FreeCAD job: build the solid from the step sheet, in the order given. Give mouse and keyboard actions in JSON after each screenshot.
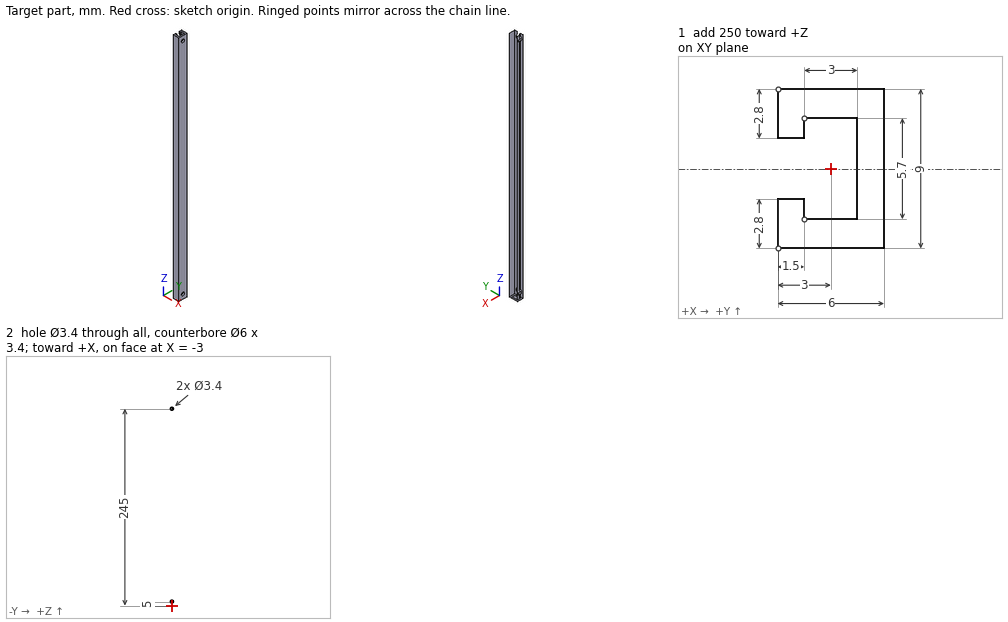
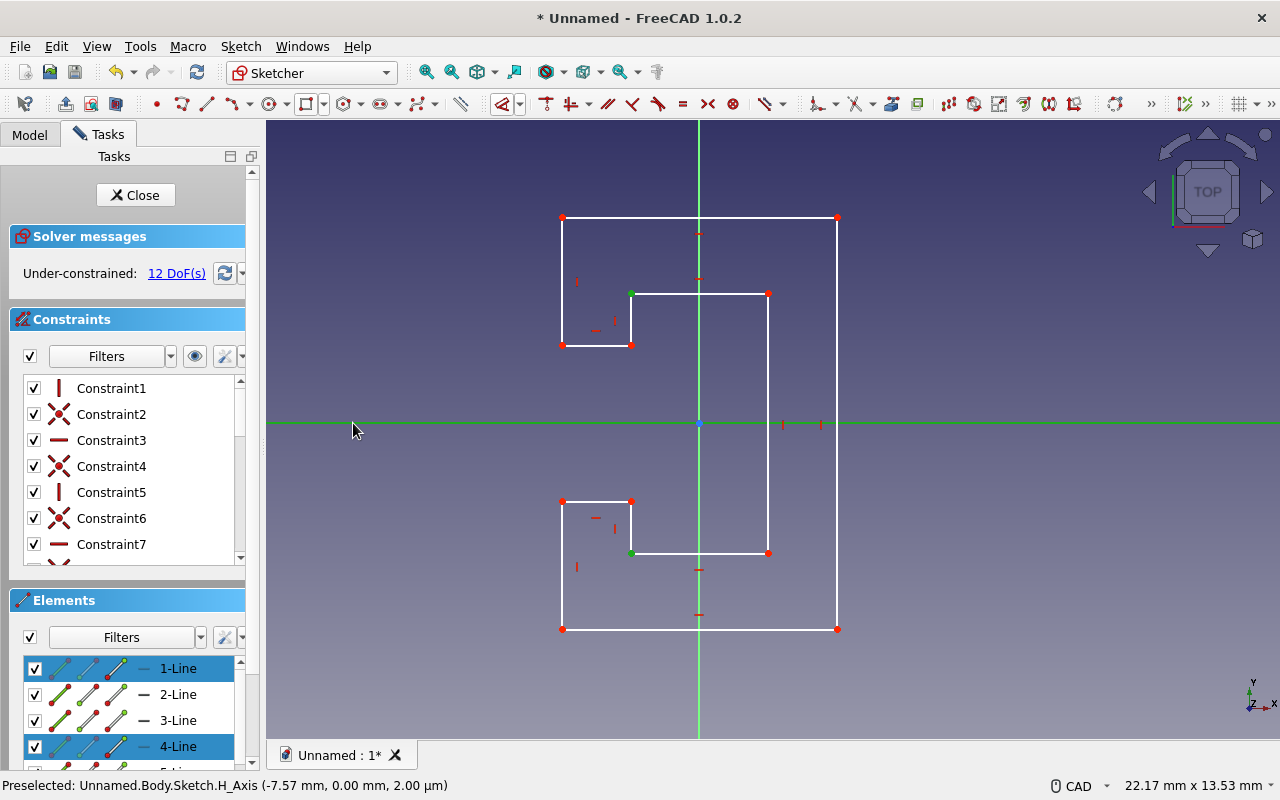
{"action": "left_click", "coordinate": [708, 104]}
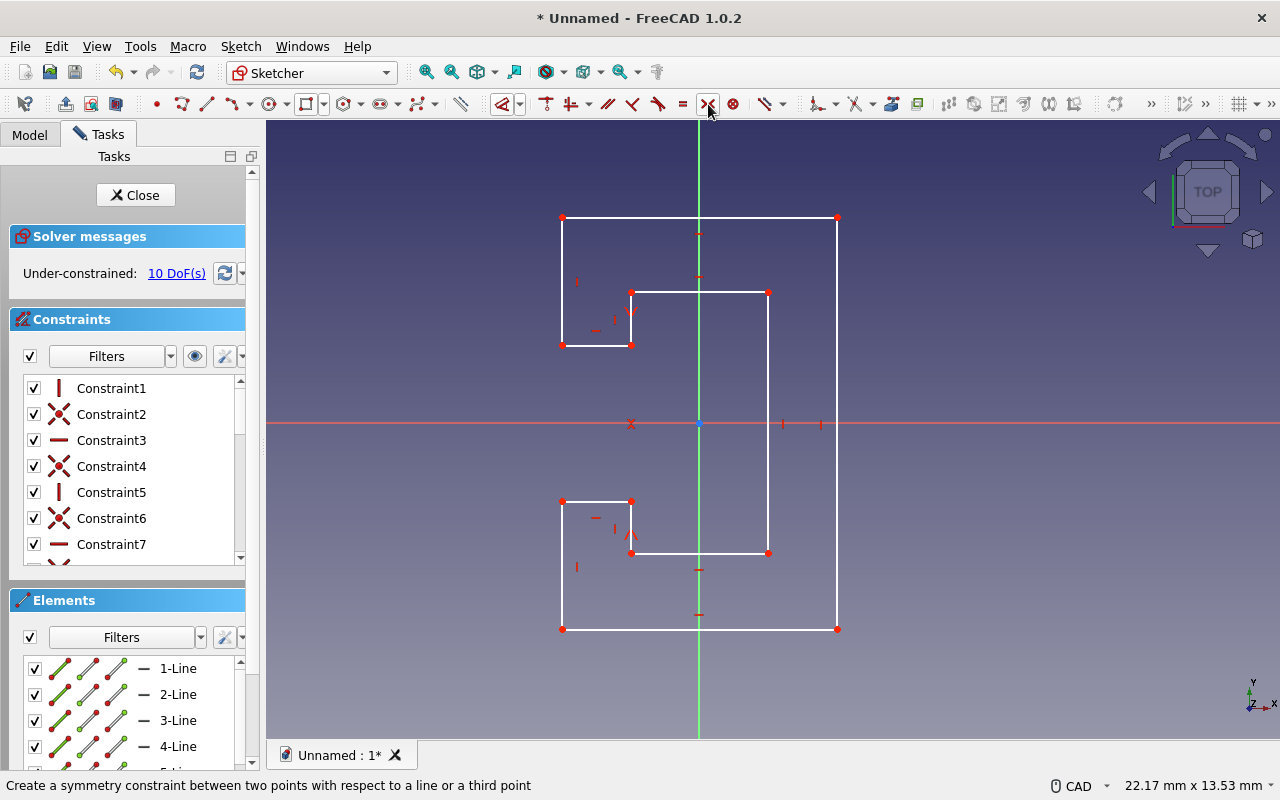
{"action": "left_click", "coordinate": [562, 630]}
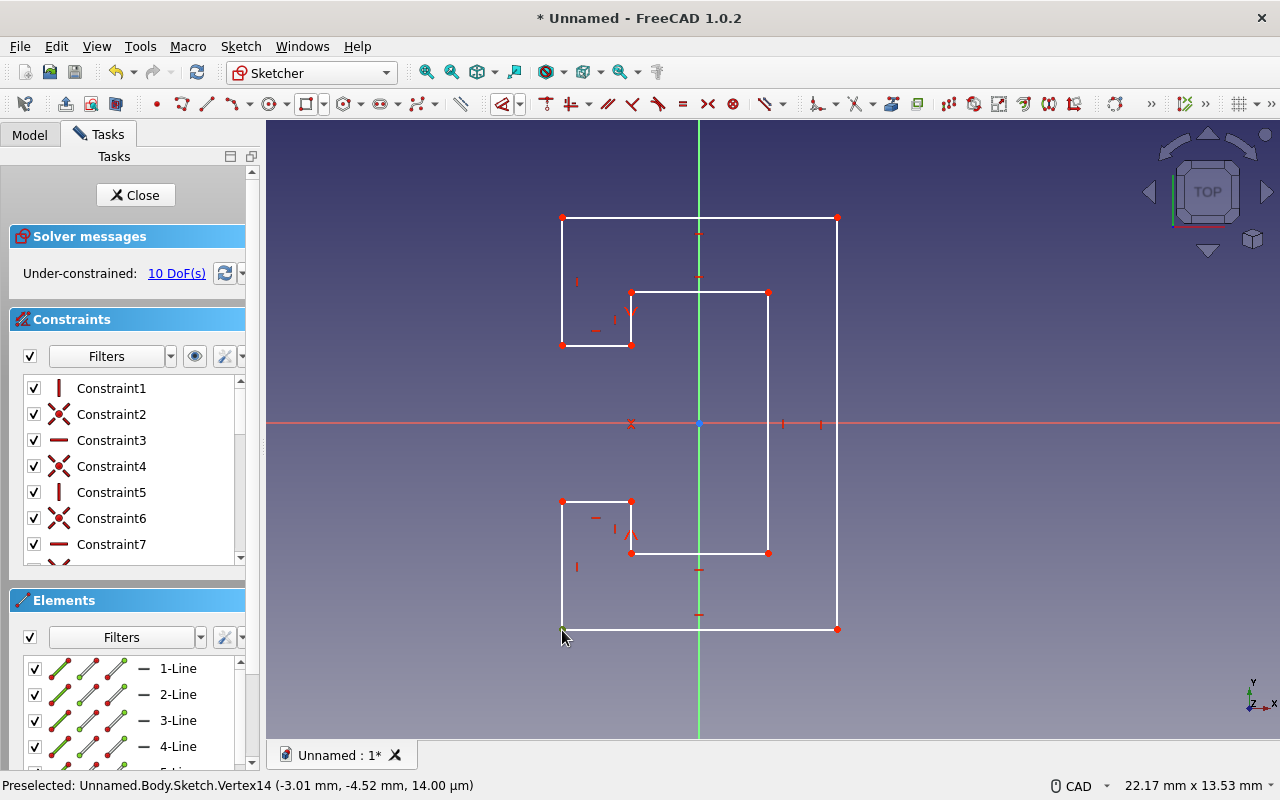
{"action": "left_click", "coordinate": [562, 218]}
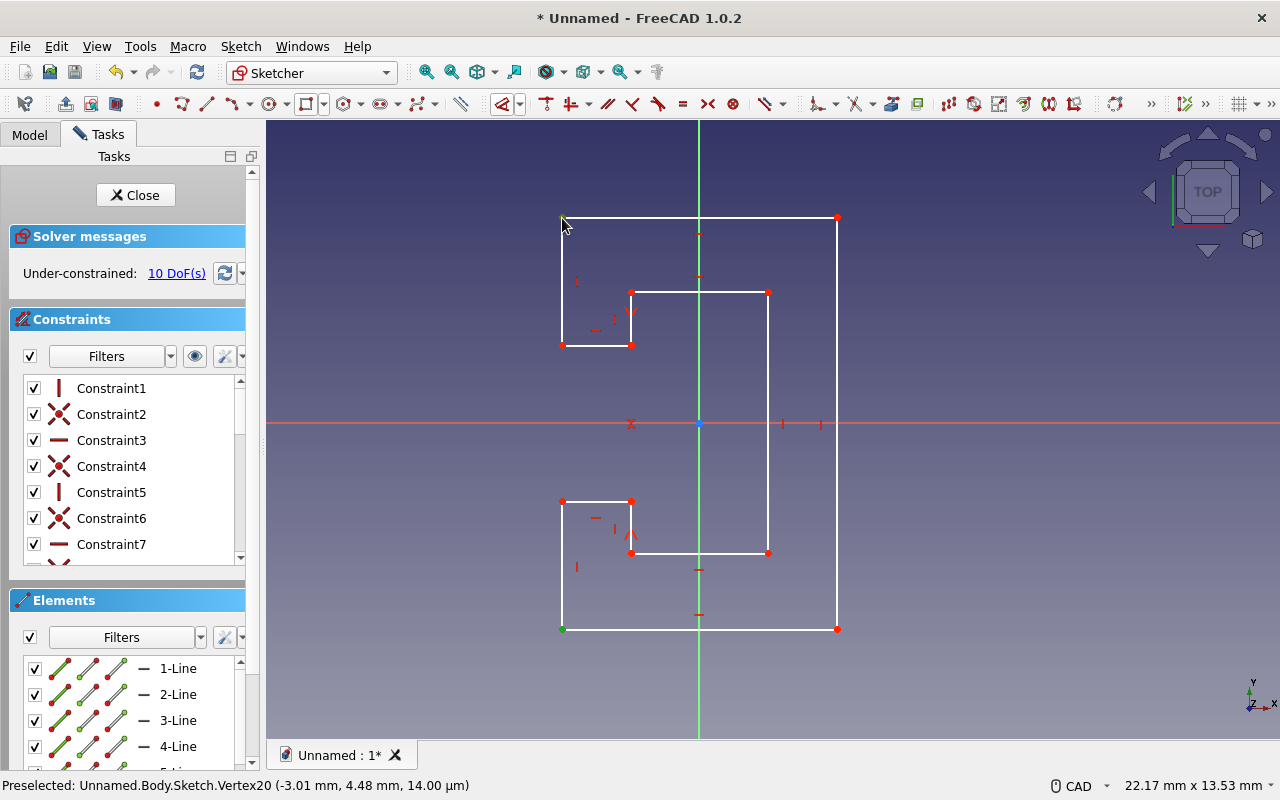
{"action": "left_click", "coordinate": [353, 423]}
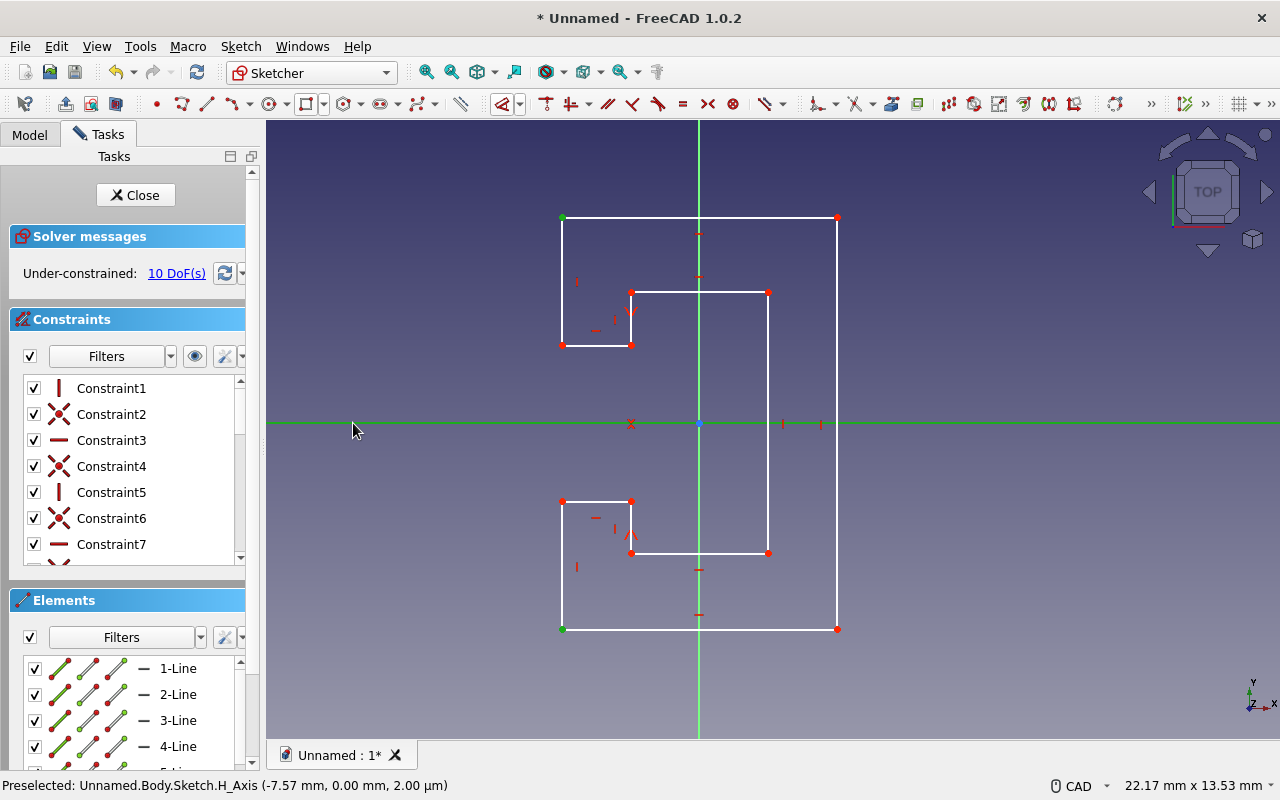
{"action": "left_click", "coordinate": [708, 104]}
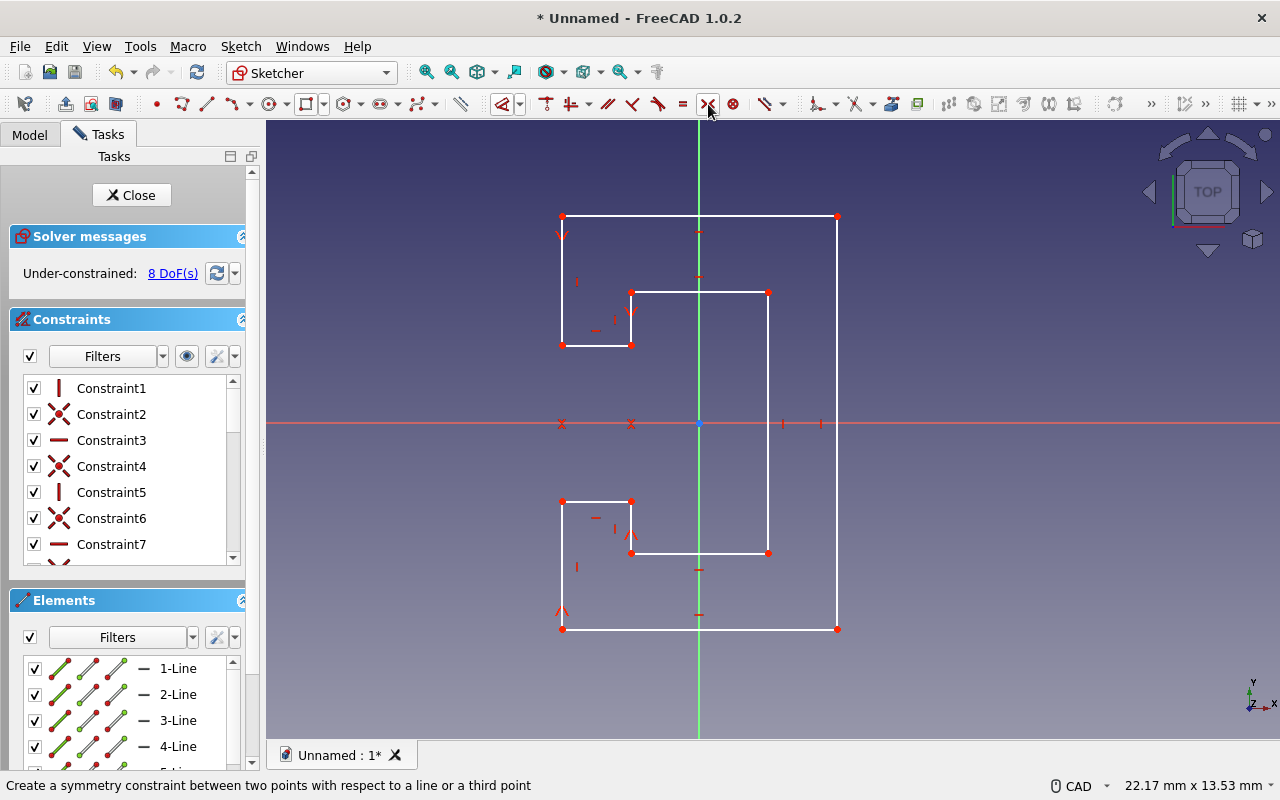
{"action": "key", "text": "d"}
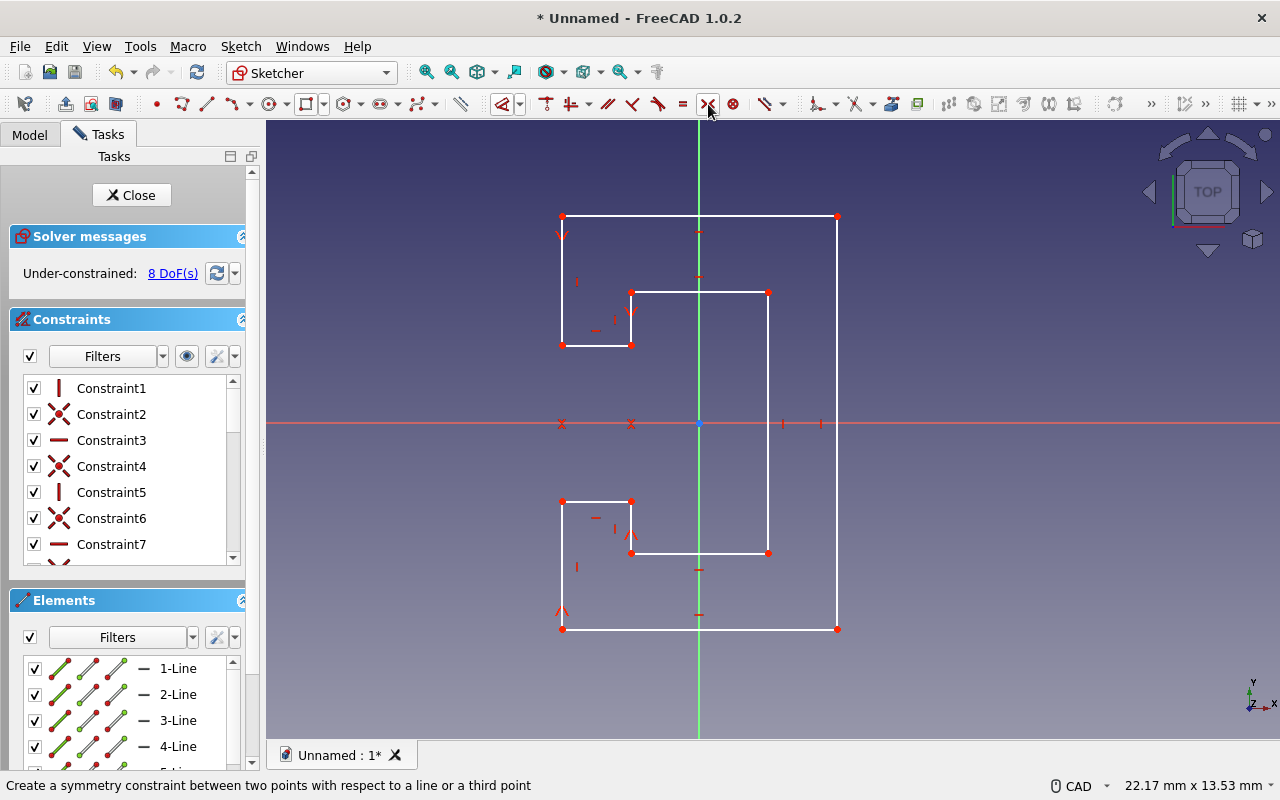
{"action": "left_click", "coordinate": [672, 292]}
{"action": "left_click", "coordinate": [668, 258]}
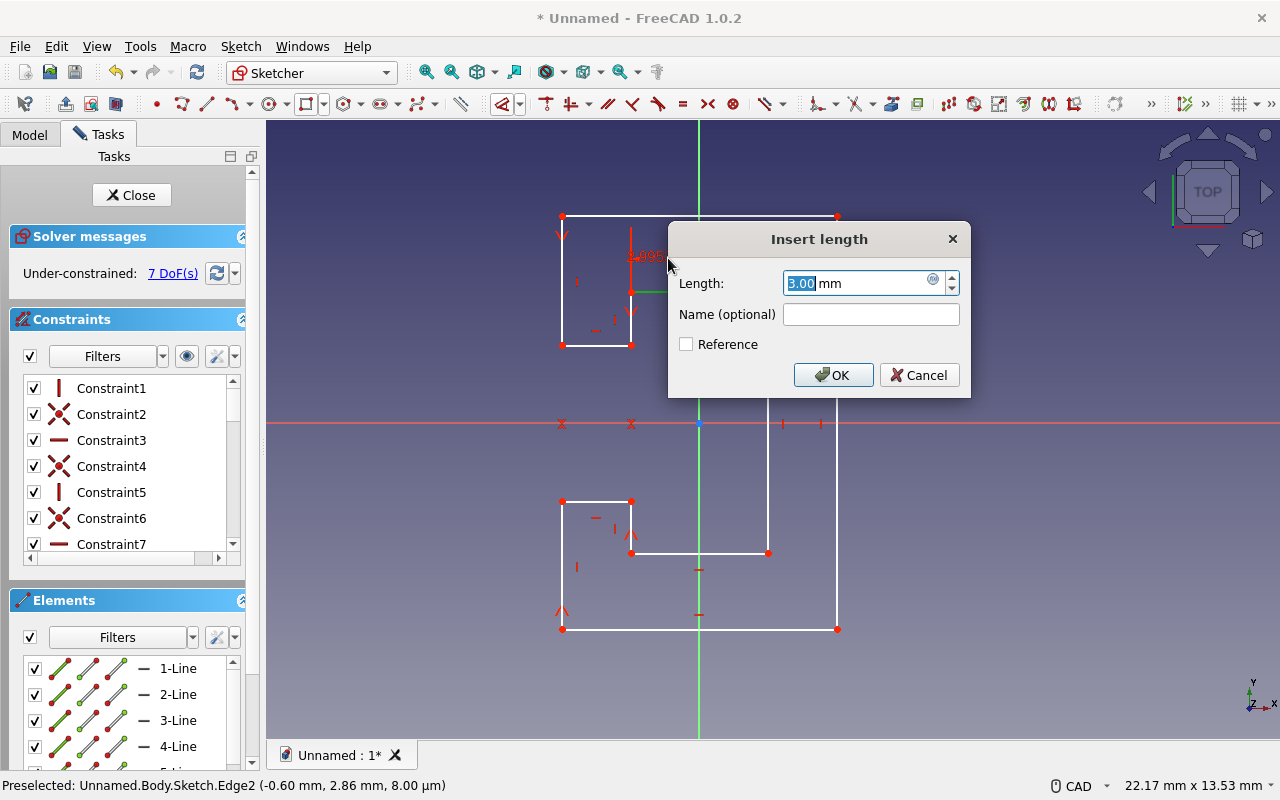
{"action": "type", "text": "3"}
{"action": "key", "text": "Return"}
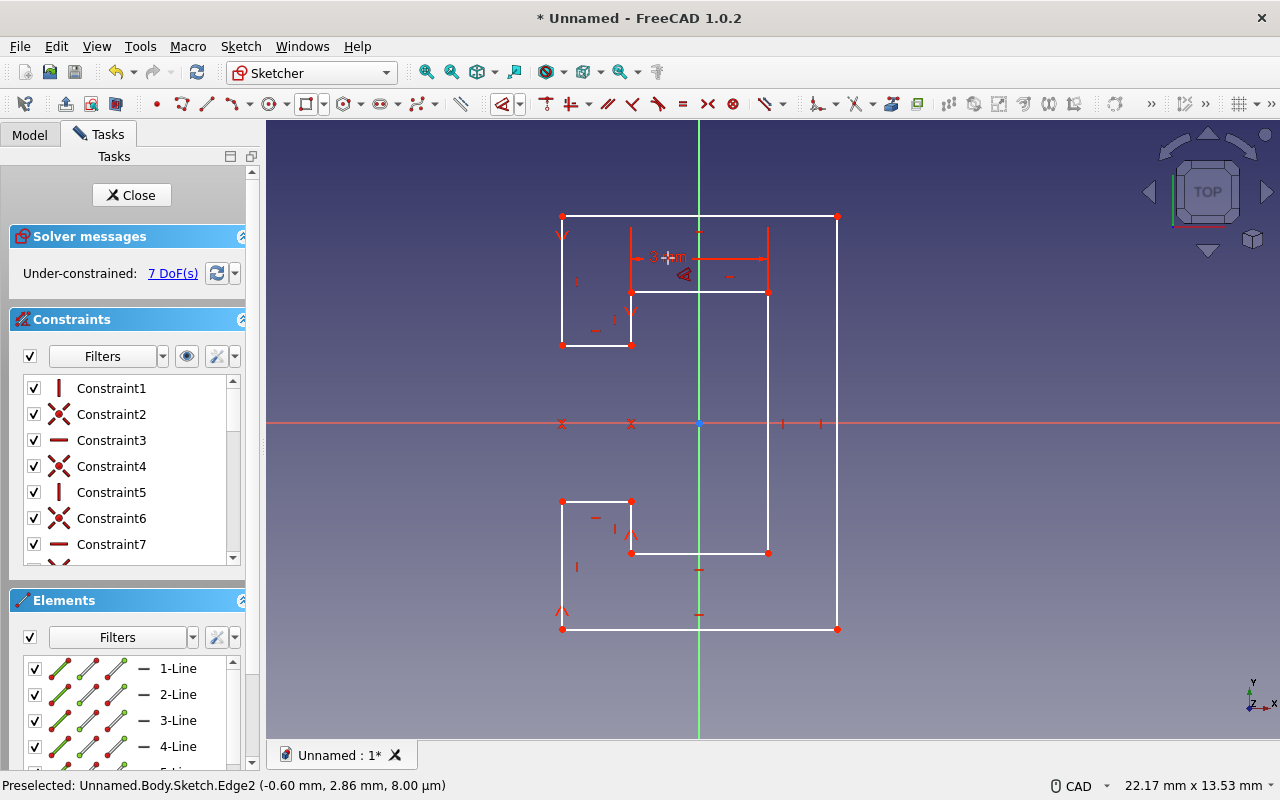
{"action": "left_click", "coordinate": [645, 630]}
{"action": "left_click", "coordinate": [636, 664]}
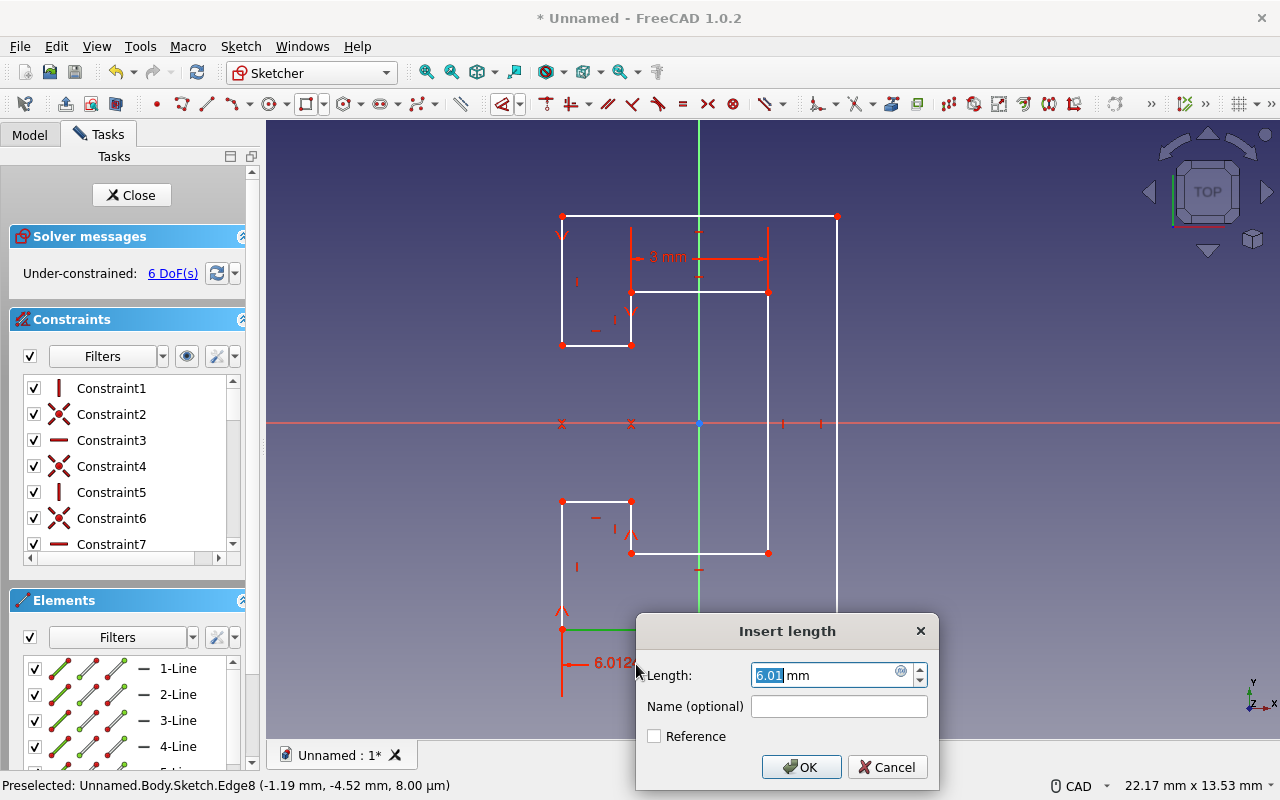
{"action": "type", "text": "6"}
{"action": "key", "text": "Return"}